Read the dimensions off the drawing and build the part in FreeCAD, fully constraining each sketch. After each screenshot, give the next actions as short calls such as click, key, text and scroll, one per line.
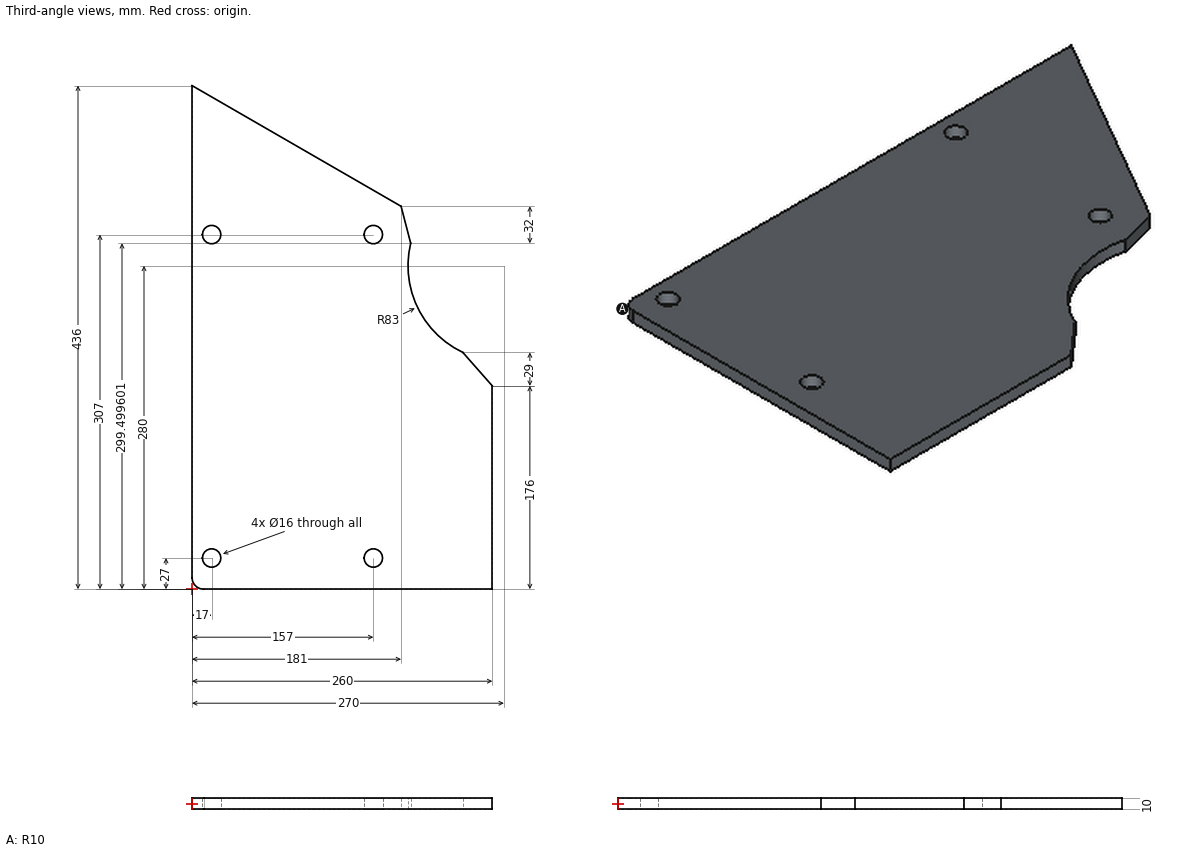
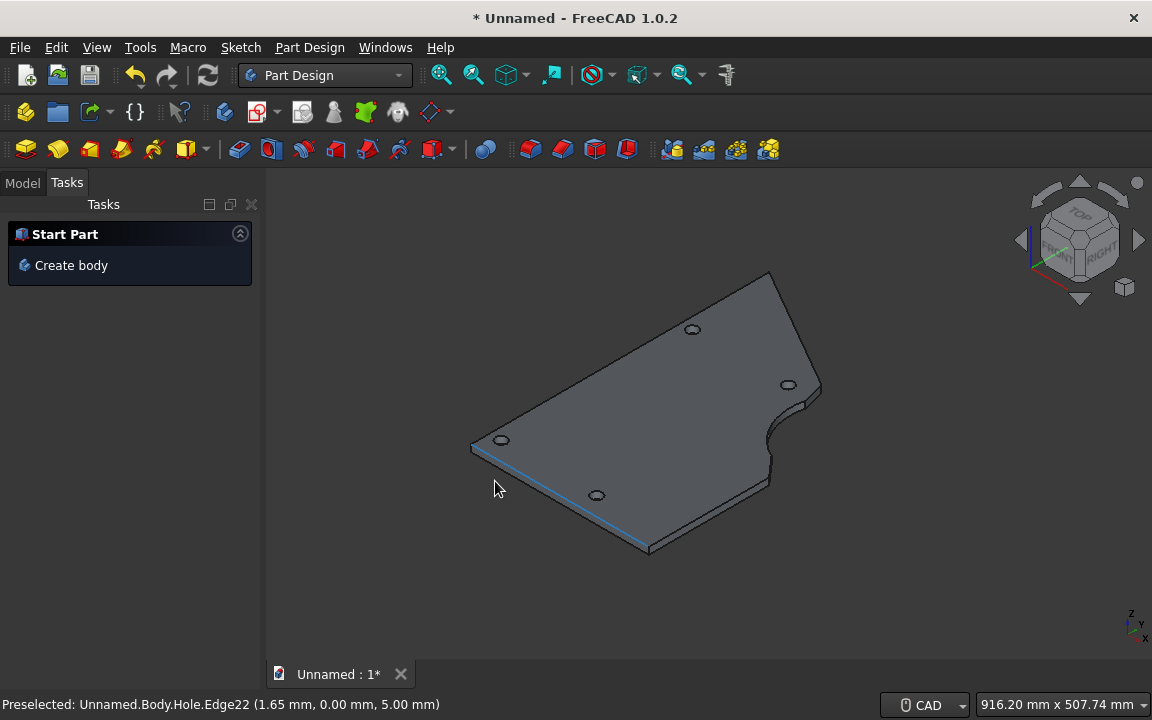
scroll(471, 447, up, 8)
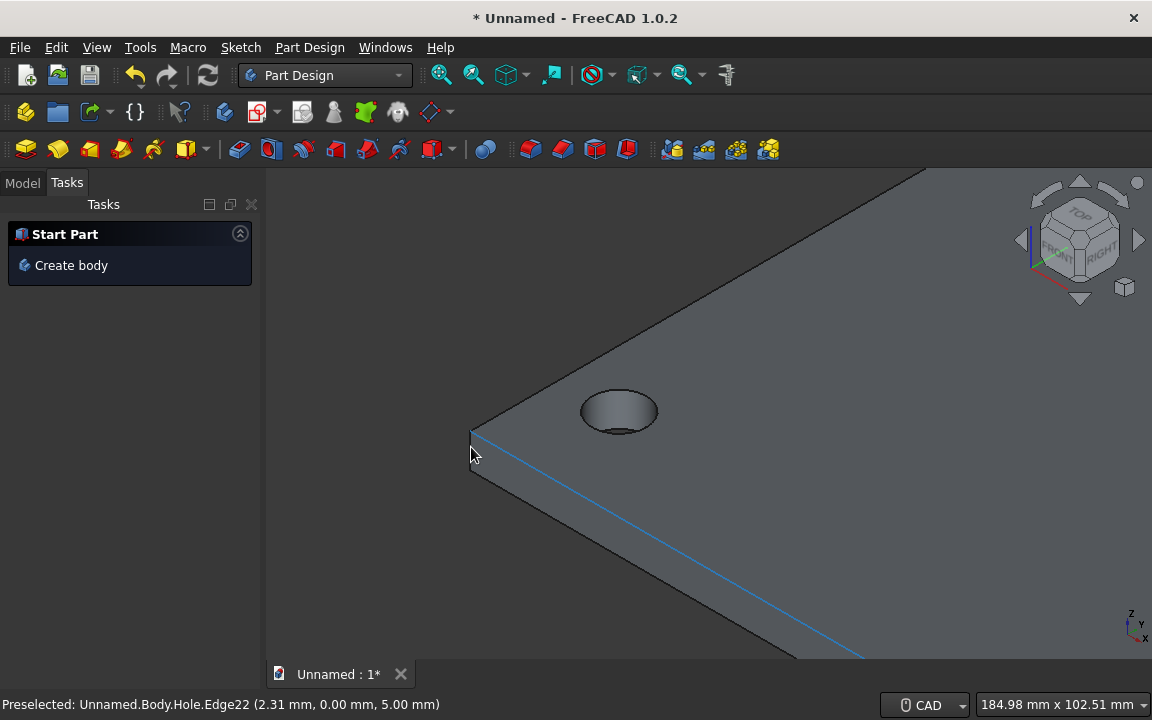
click(442, 76)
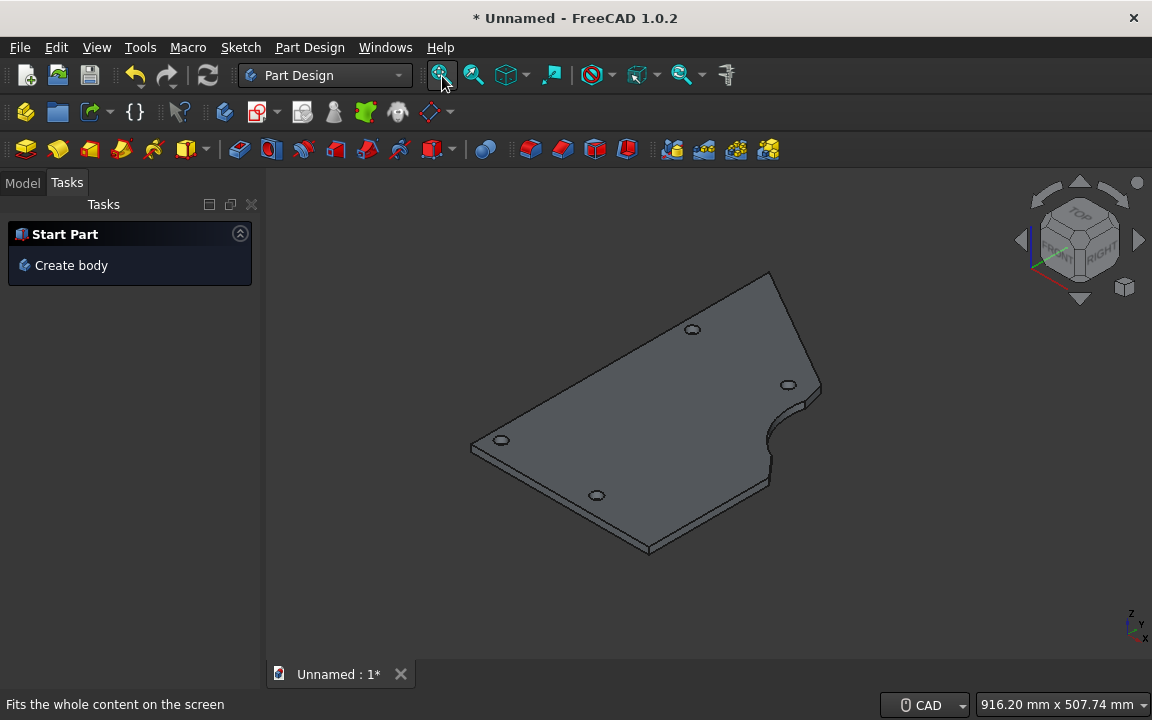
key(2)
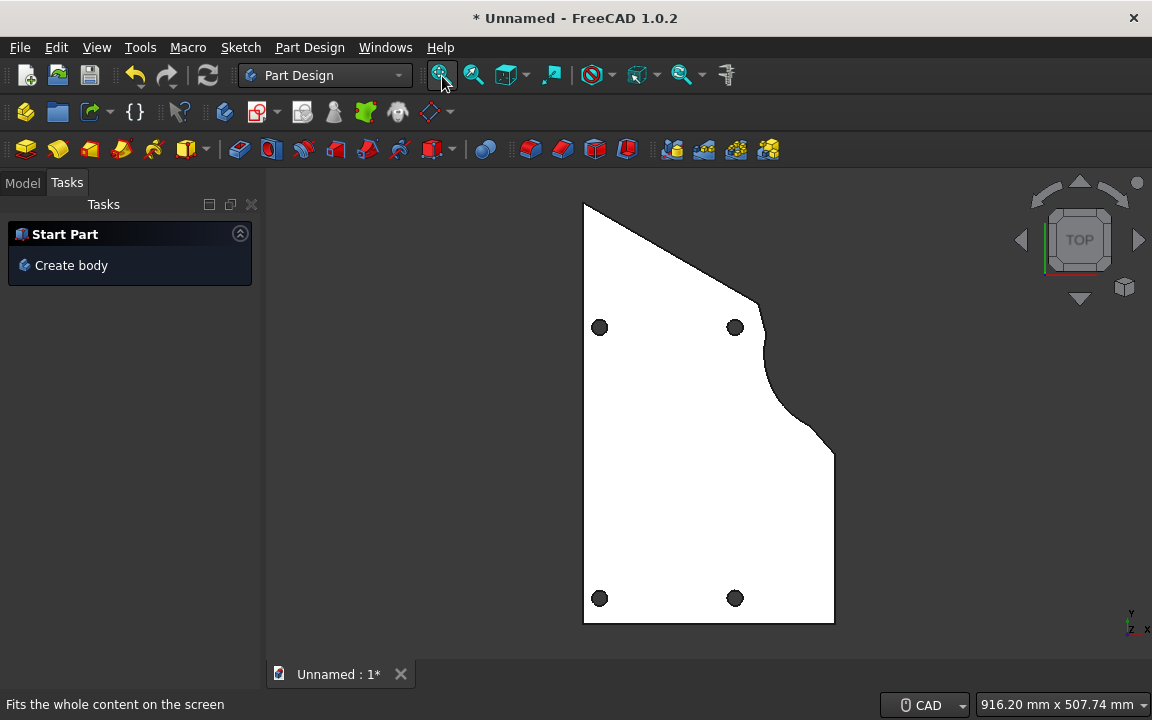
scroll(583, 623, up, 8)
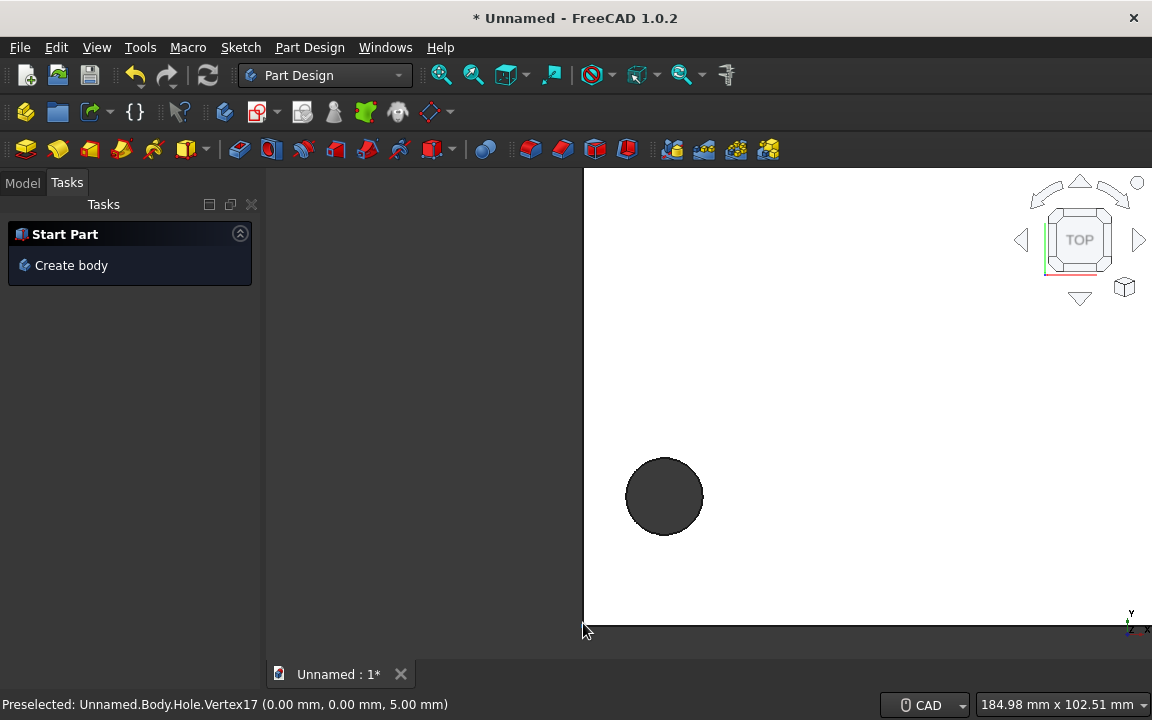
key(v)
key(f)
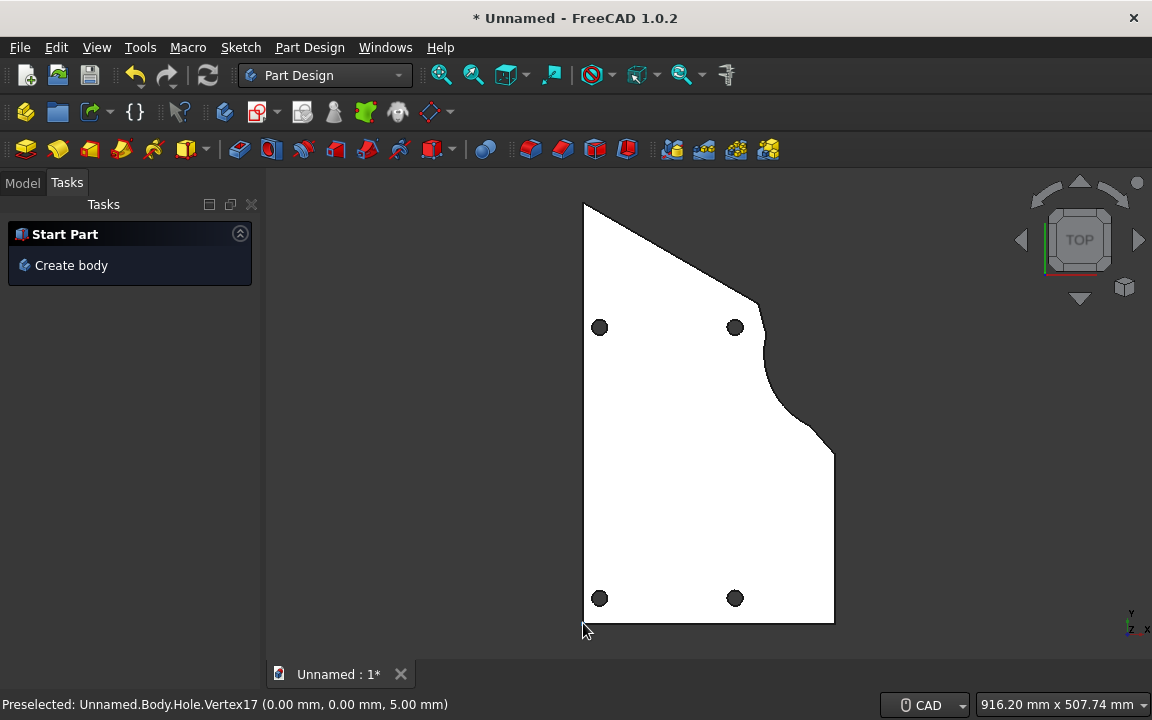
key(1)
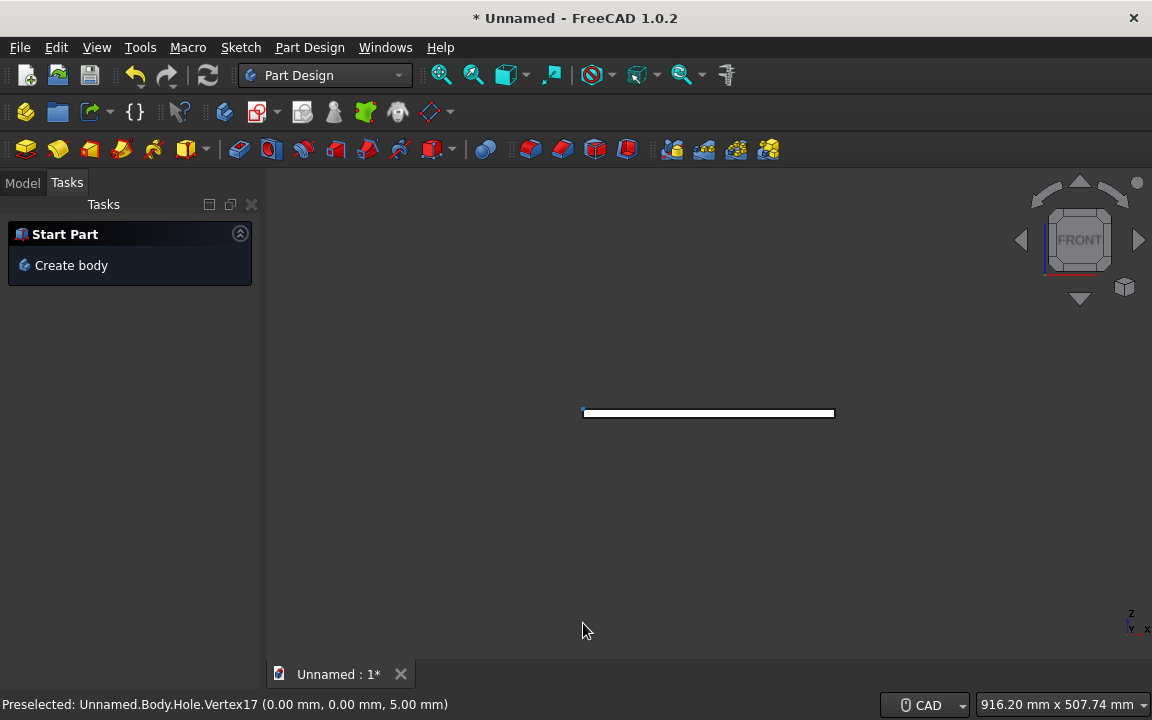
key(v)
key(f)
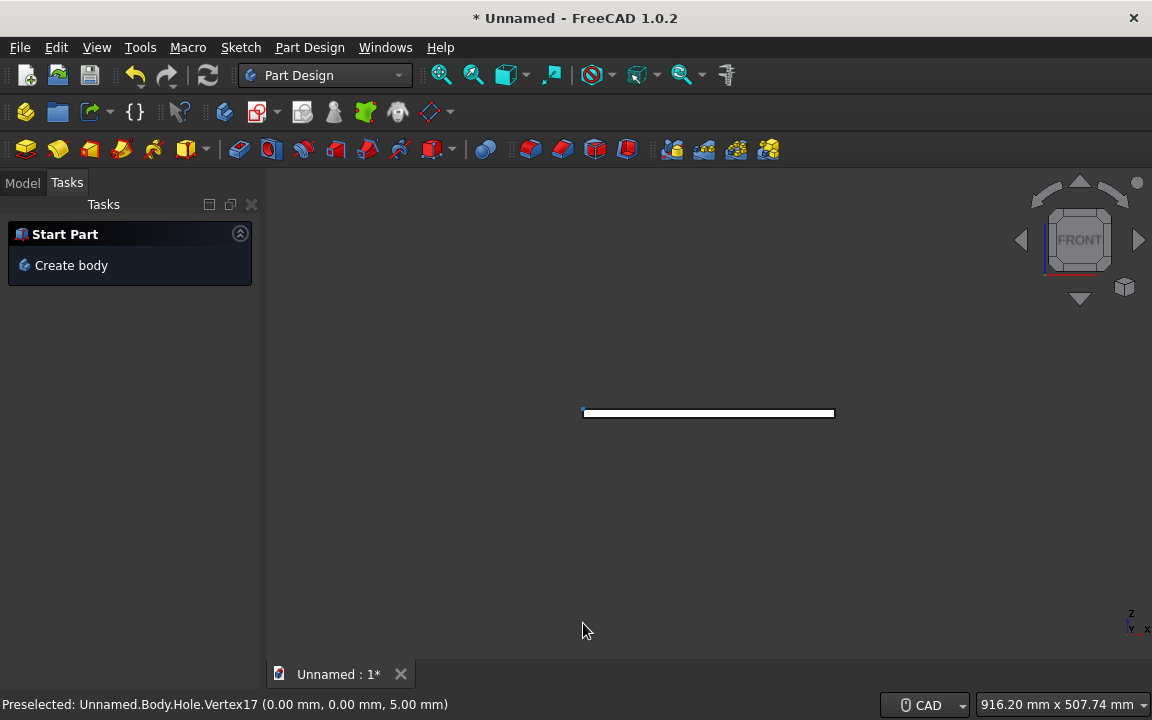
scroll(583, 413, up, 8)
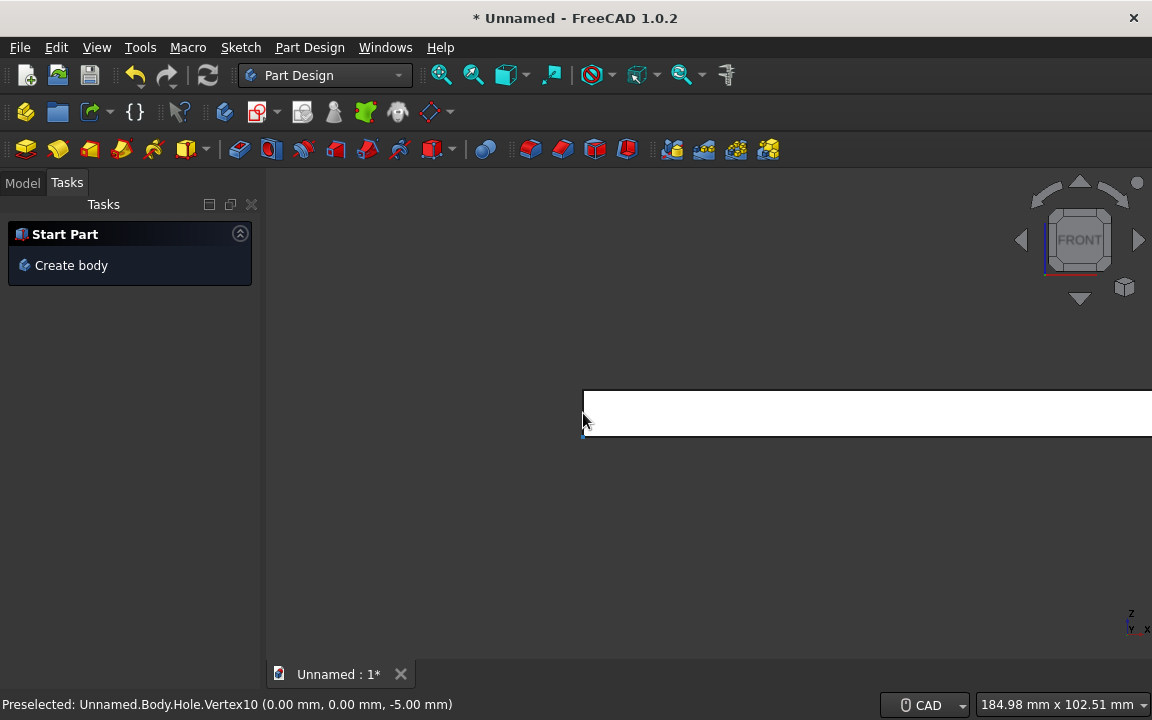
click(583, 413)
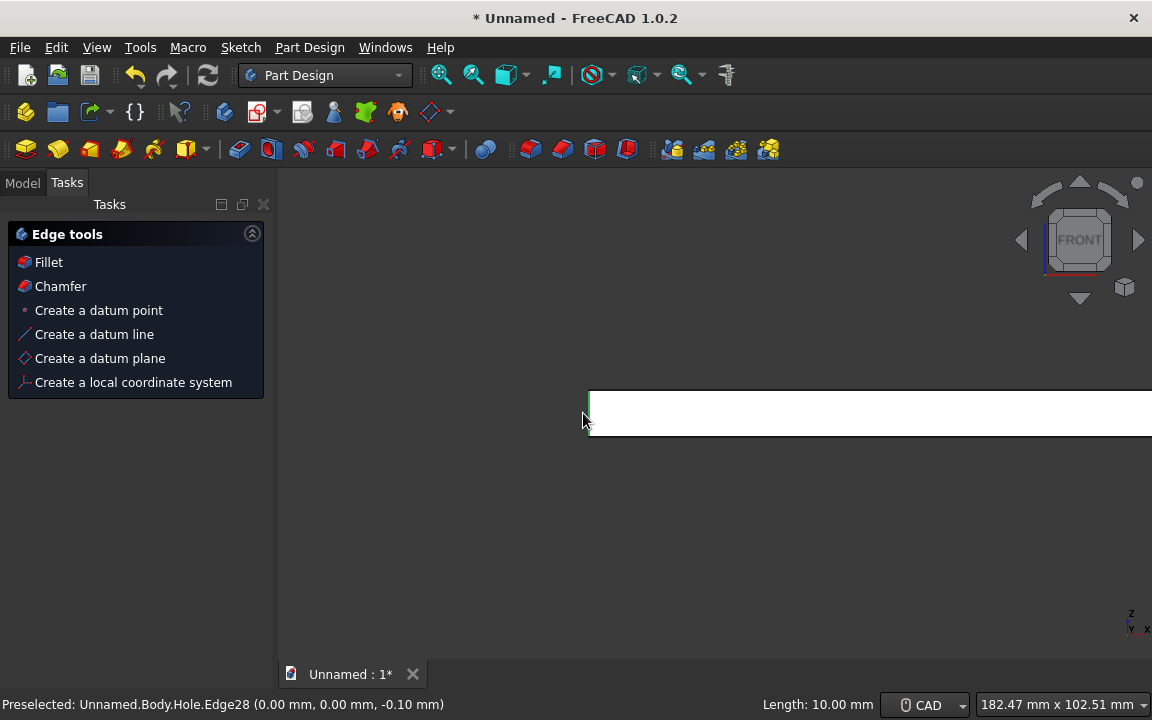
click(532, 150)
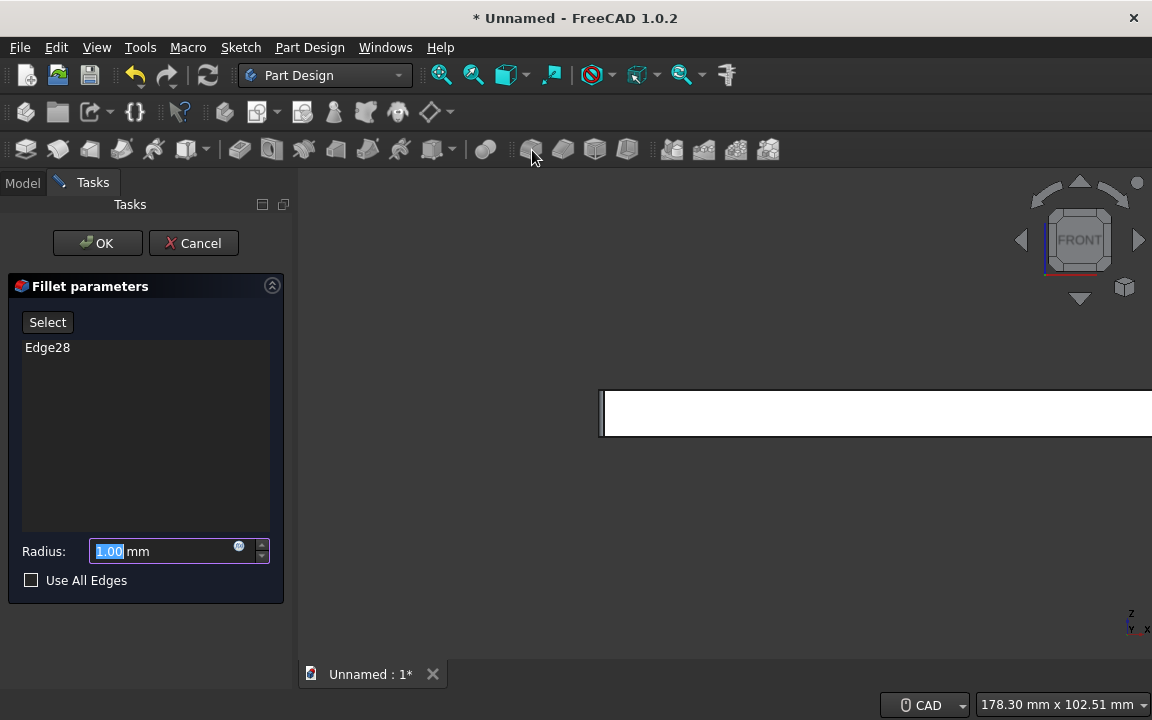
text(10)
key(Tab)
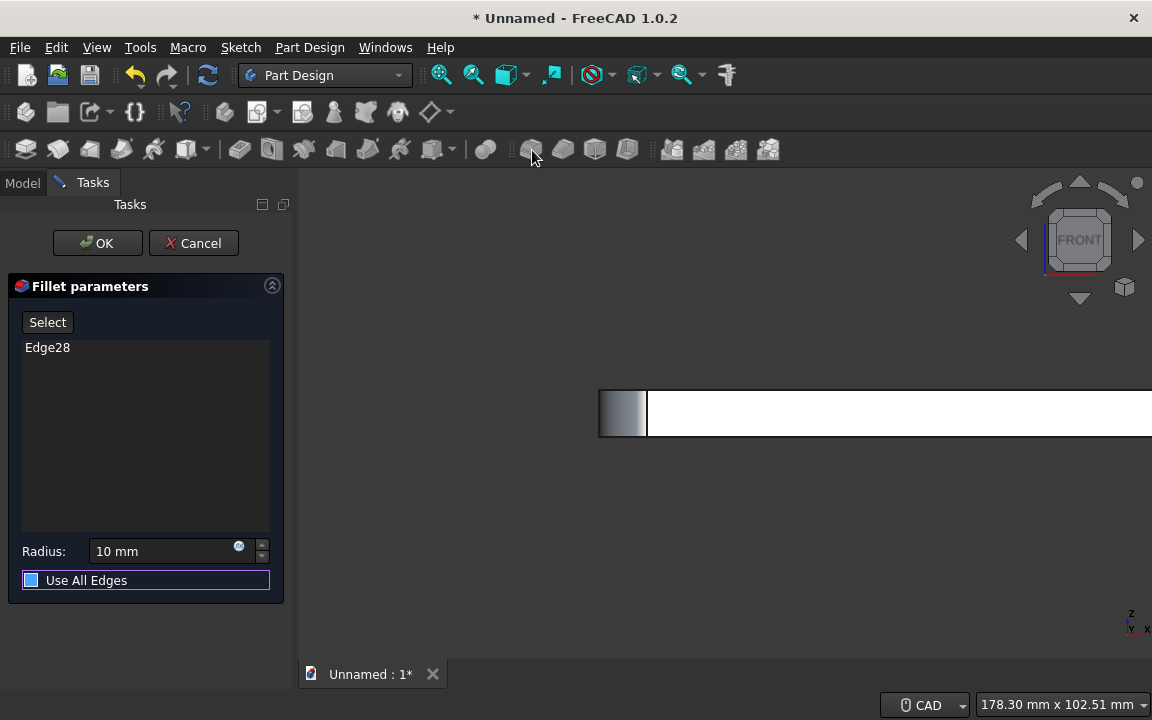
click(98, 243)